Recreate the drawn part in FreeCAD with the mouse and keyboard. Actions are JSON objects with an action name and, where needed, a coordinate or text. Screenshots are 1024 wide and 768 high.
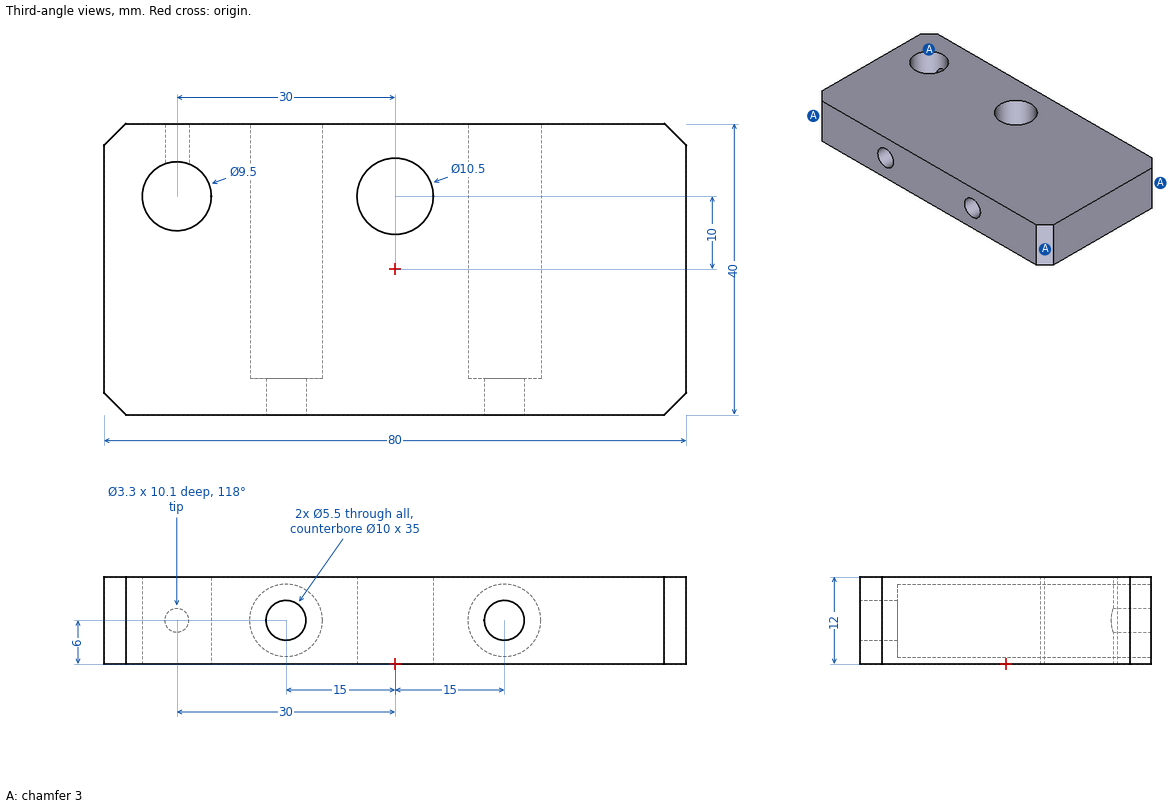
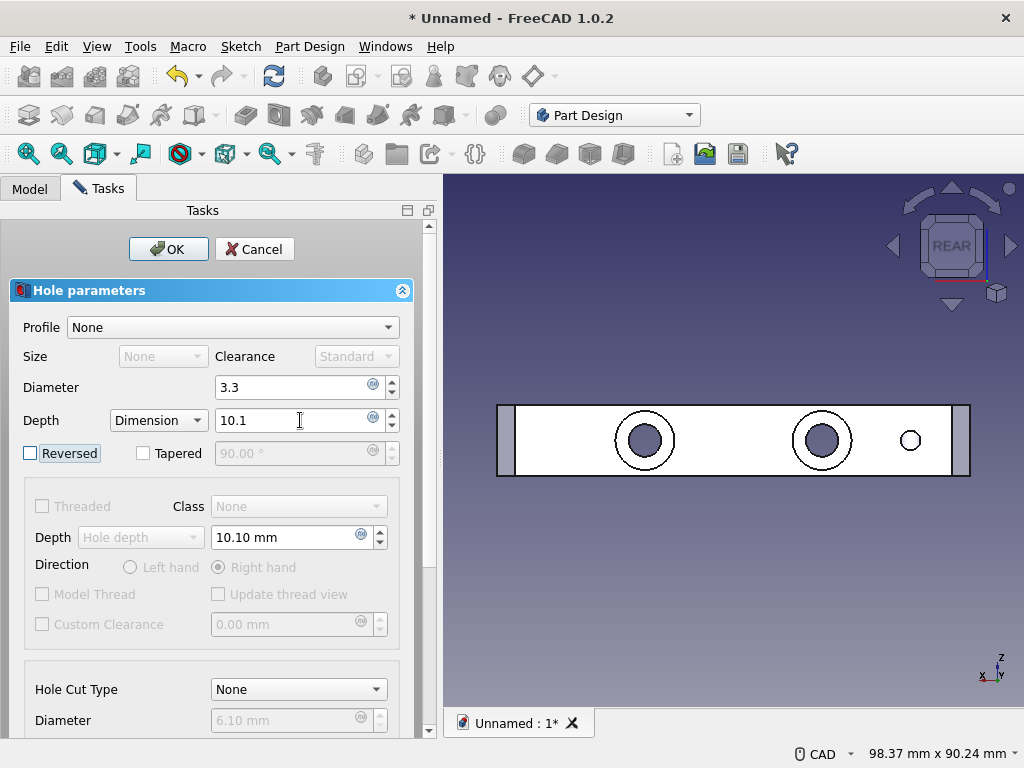
{"action": "left_click", "coordinate": [169, 249]}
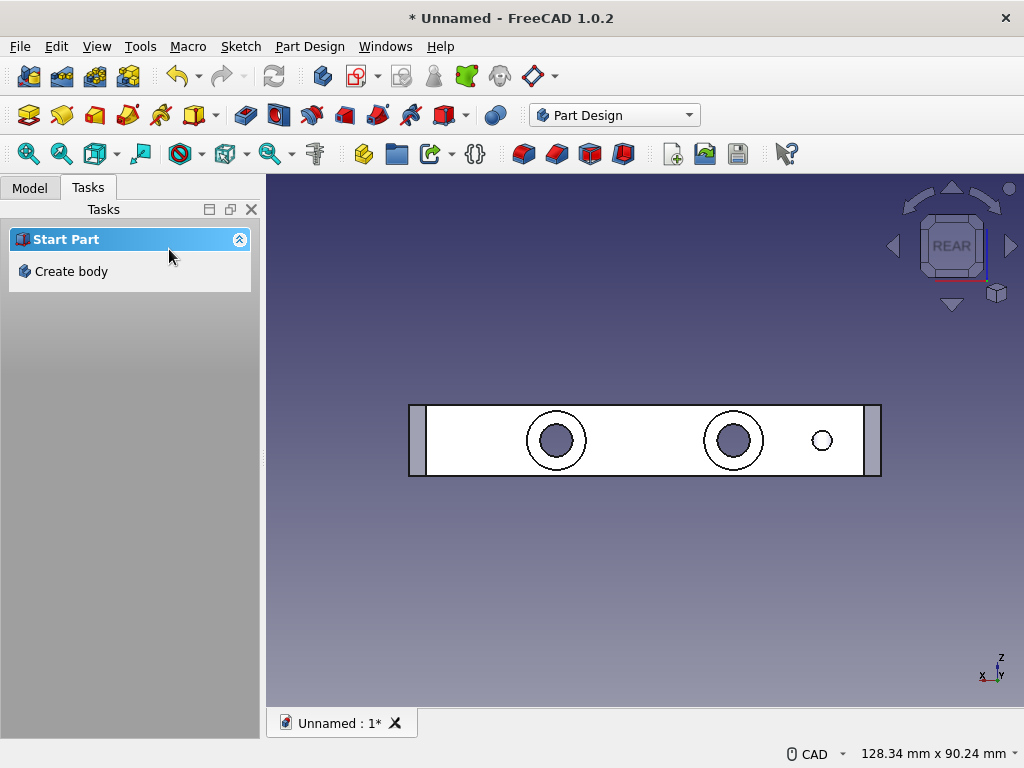
{"action": "key", "text": "0"}